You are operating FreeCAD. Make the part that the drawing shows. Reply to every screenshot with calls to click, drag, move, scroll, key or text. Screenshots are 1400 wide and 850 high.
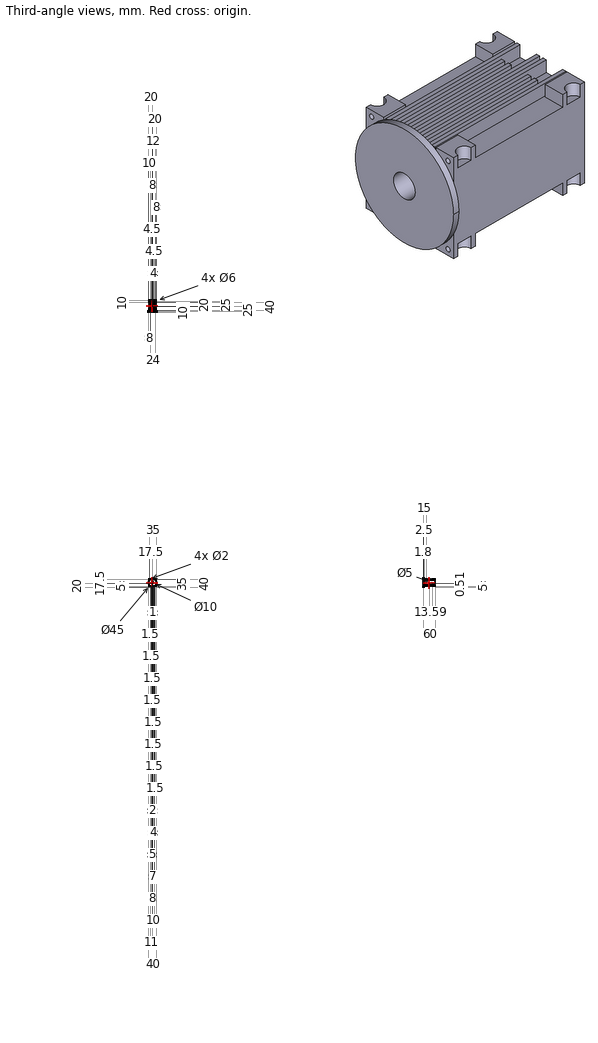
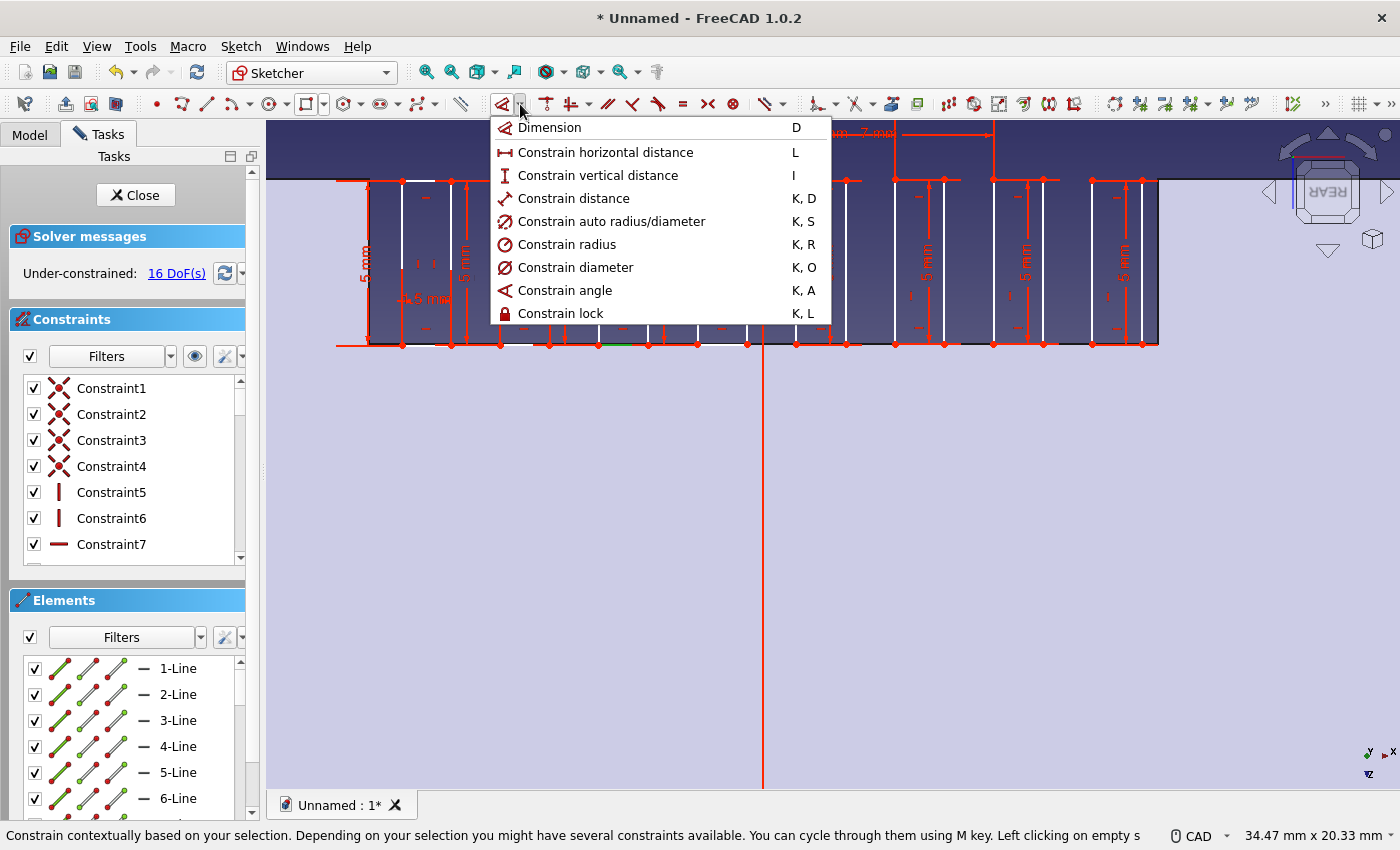
click(661, 152)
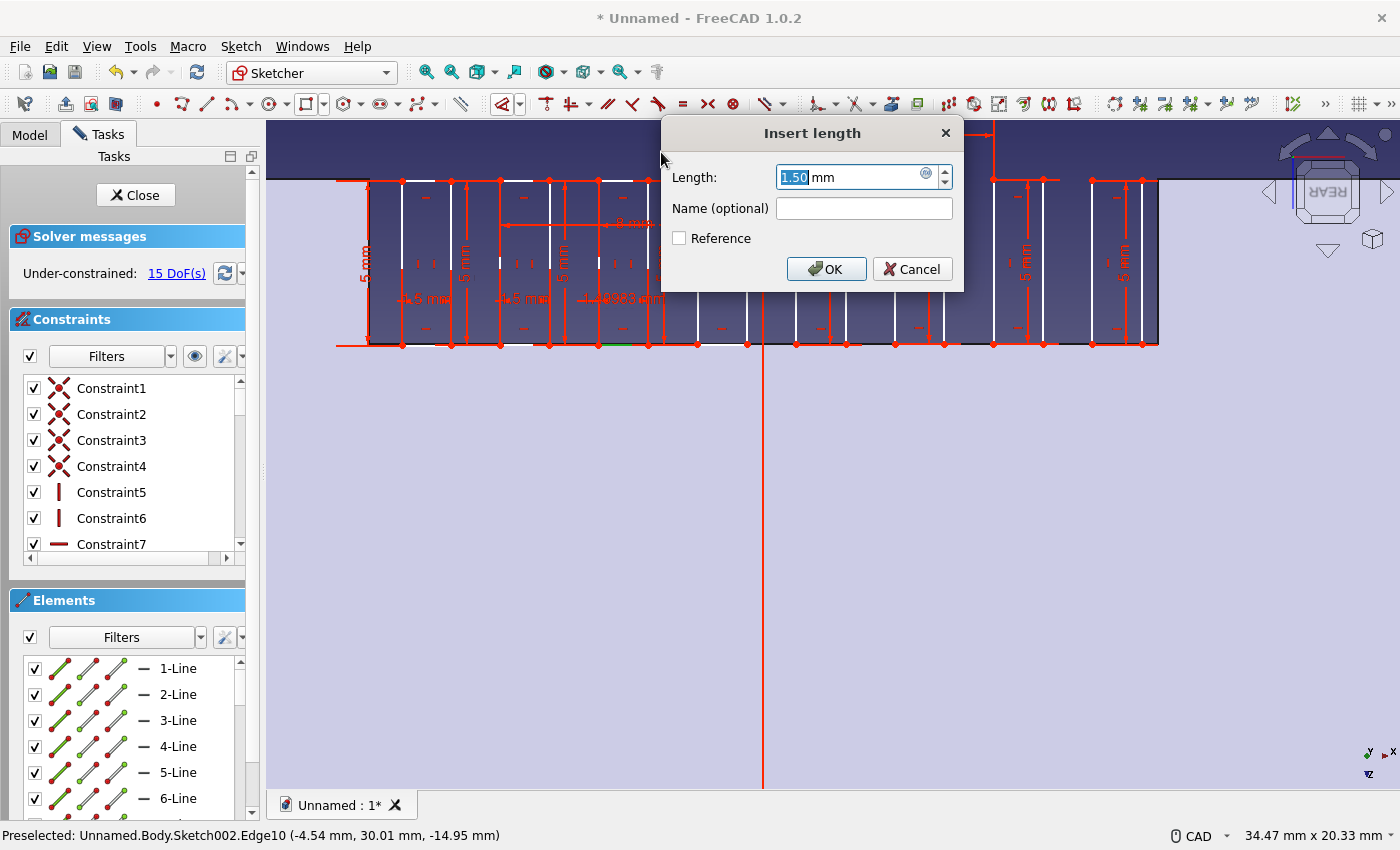
text(1.5)
key(Return)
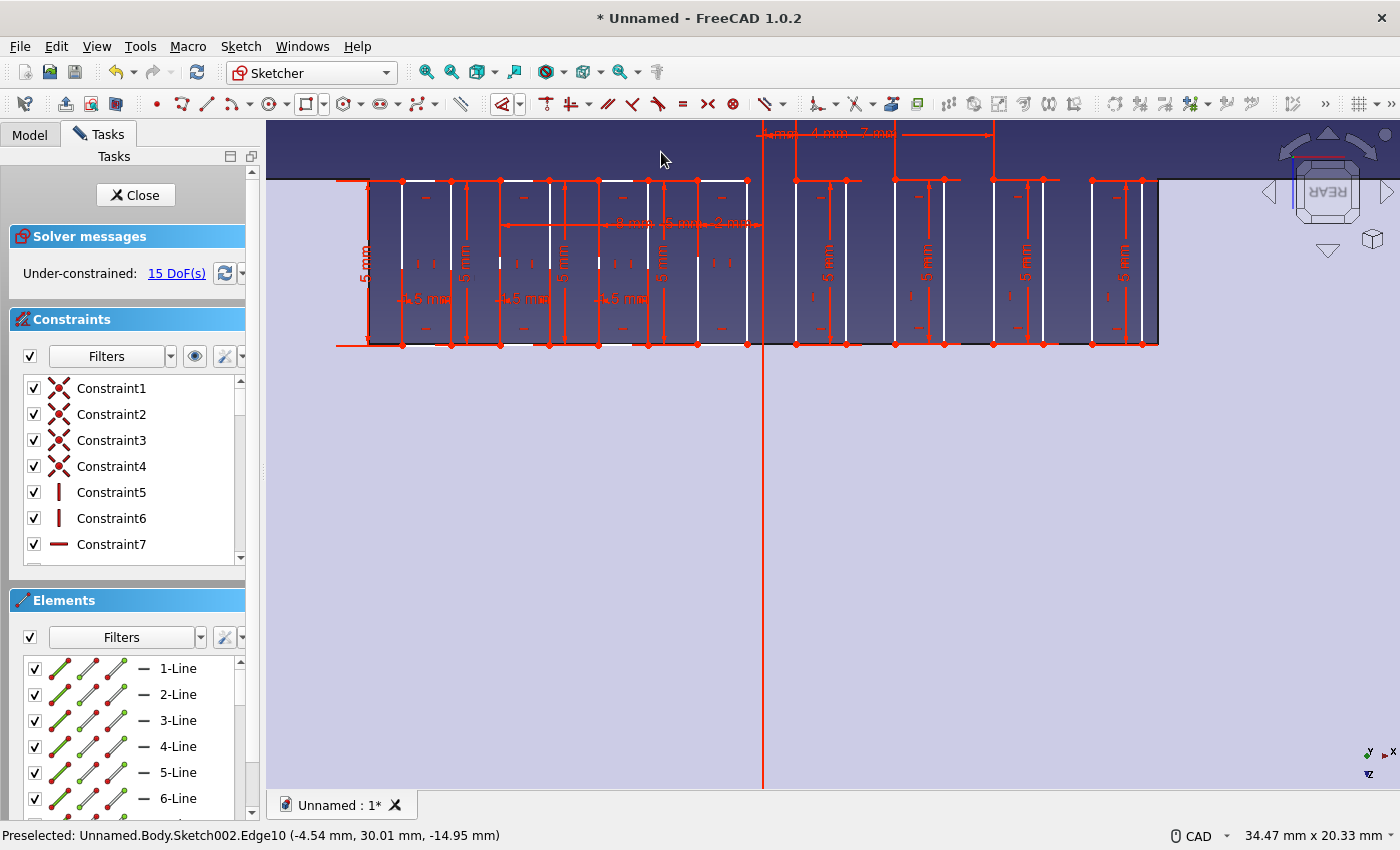
click(712, 345)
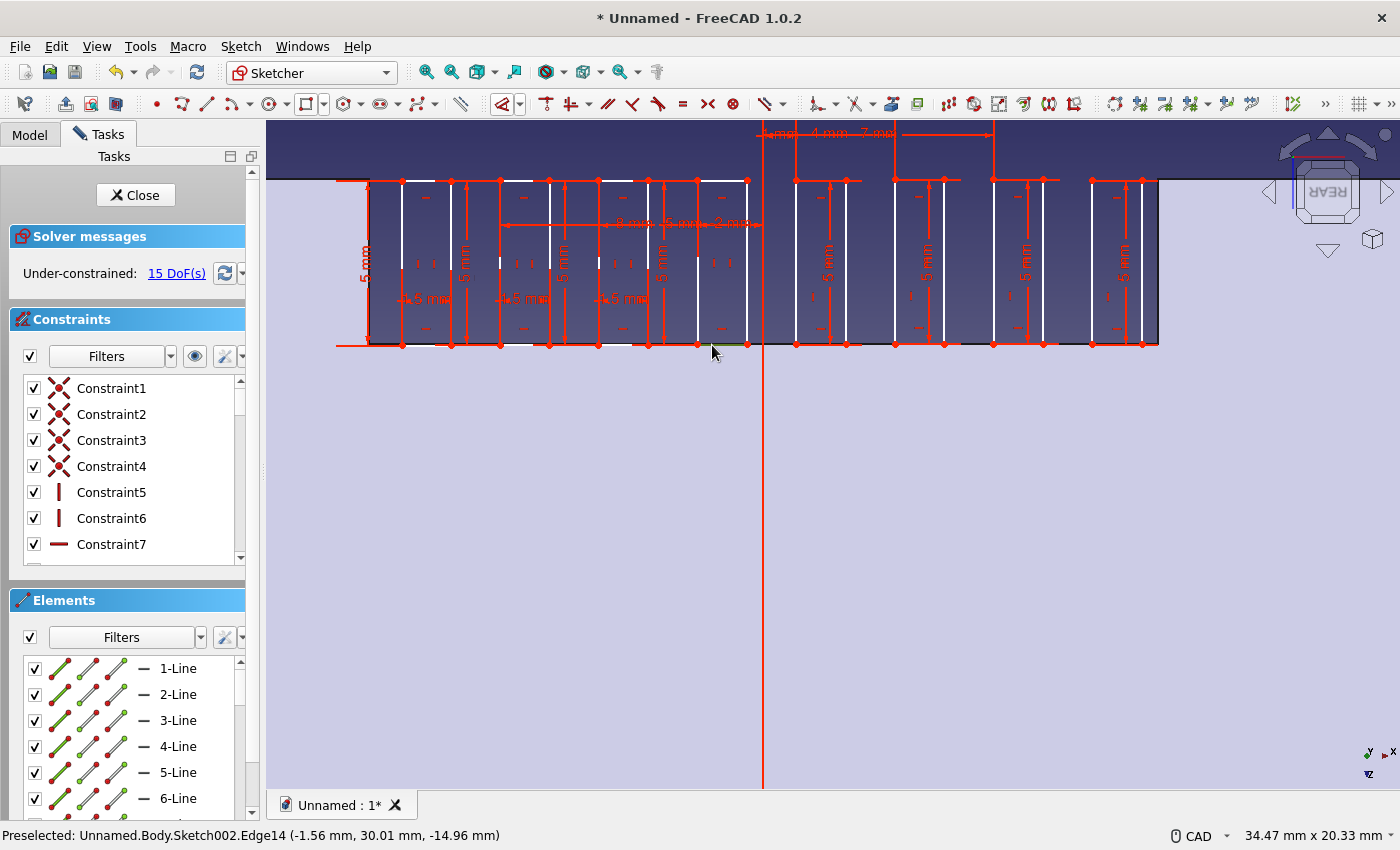
click(520, 104)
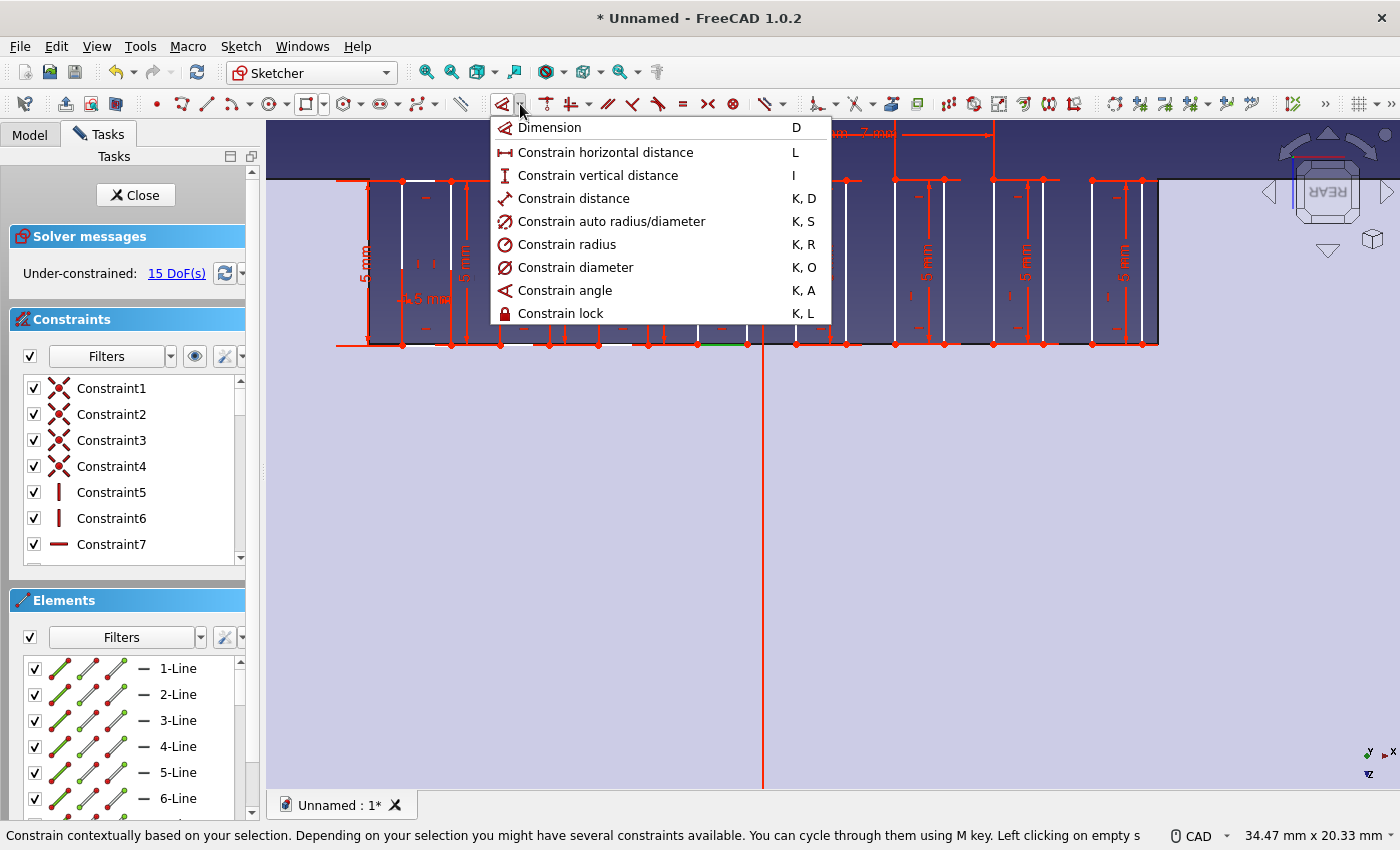
click(661, 152)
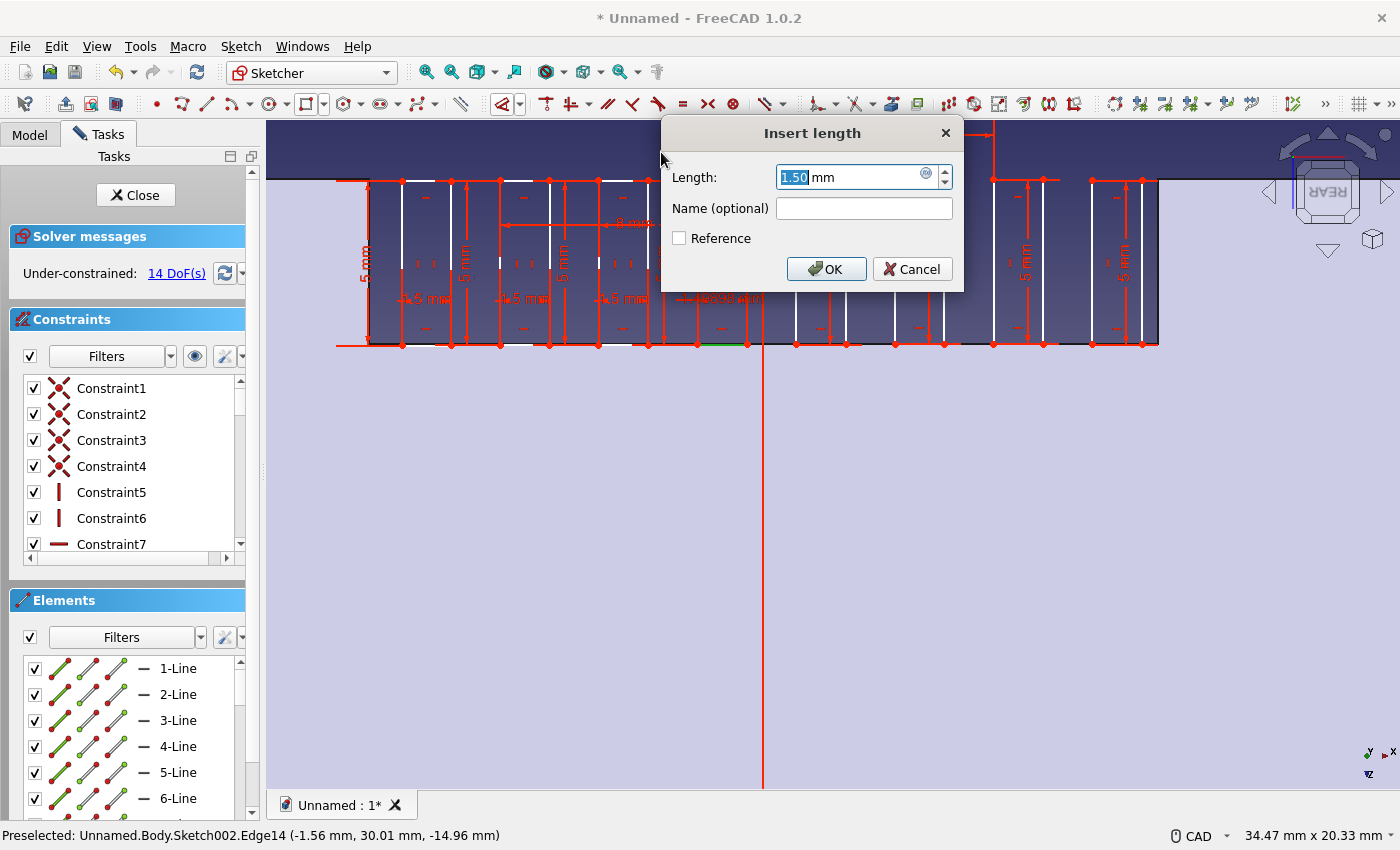
text(1.5)
key(Return)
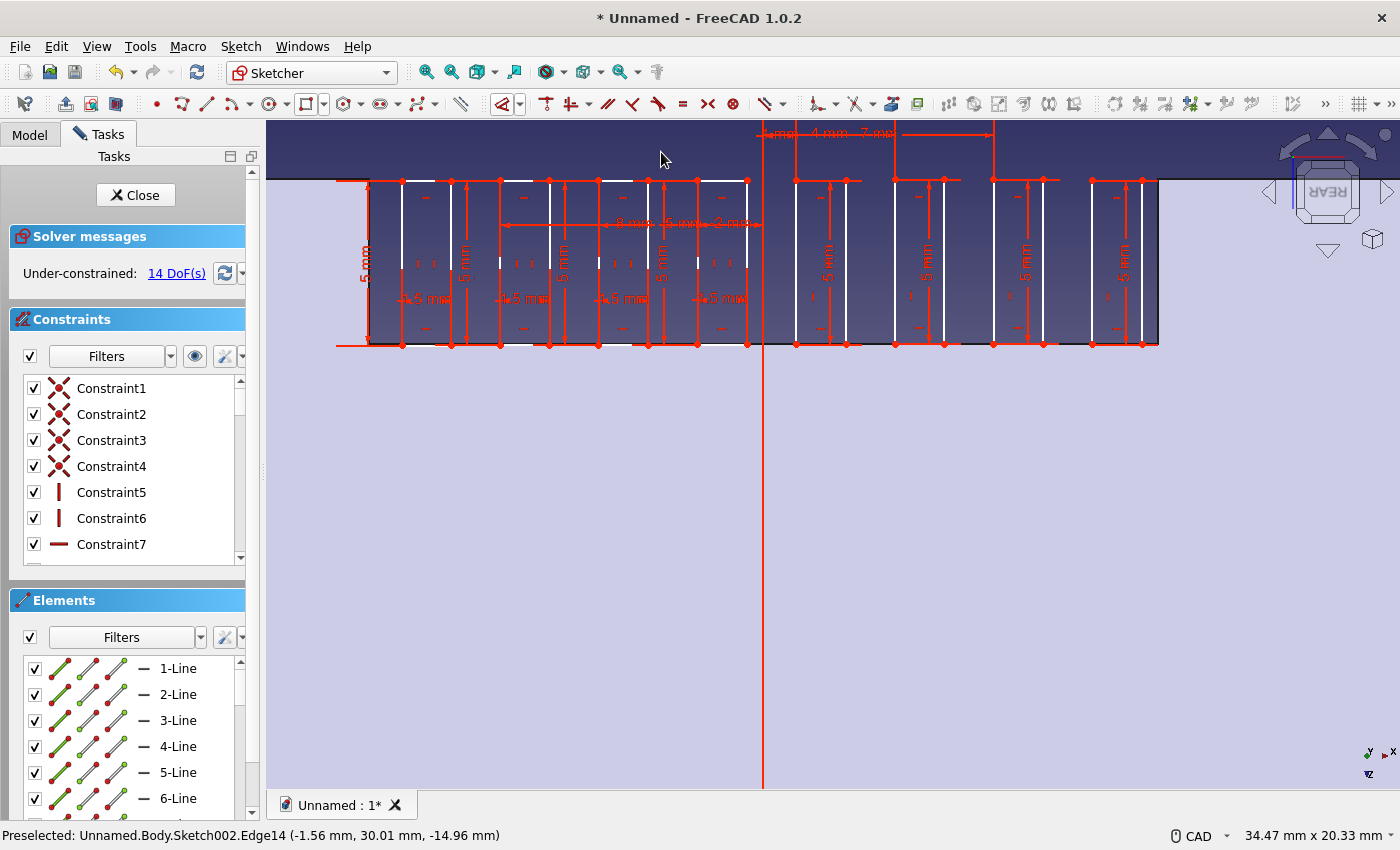
click(811, 345)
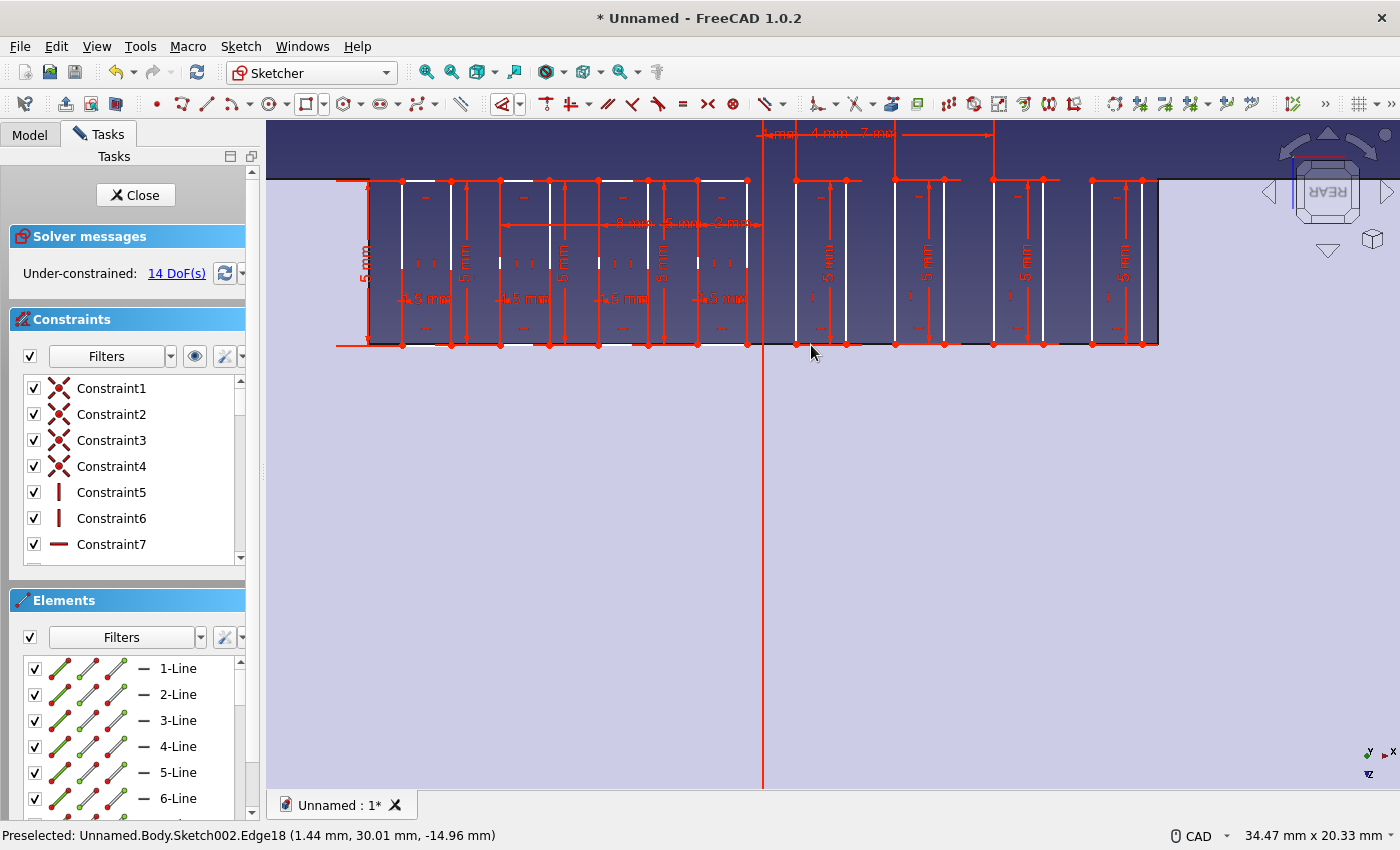
key(l)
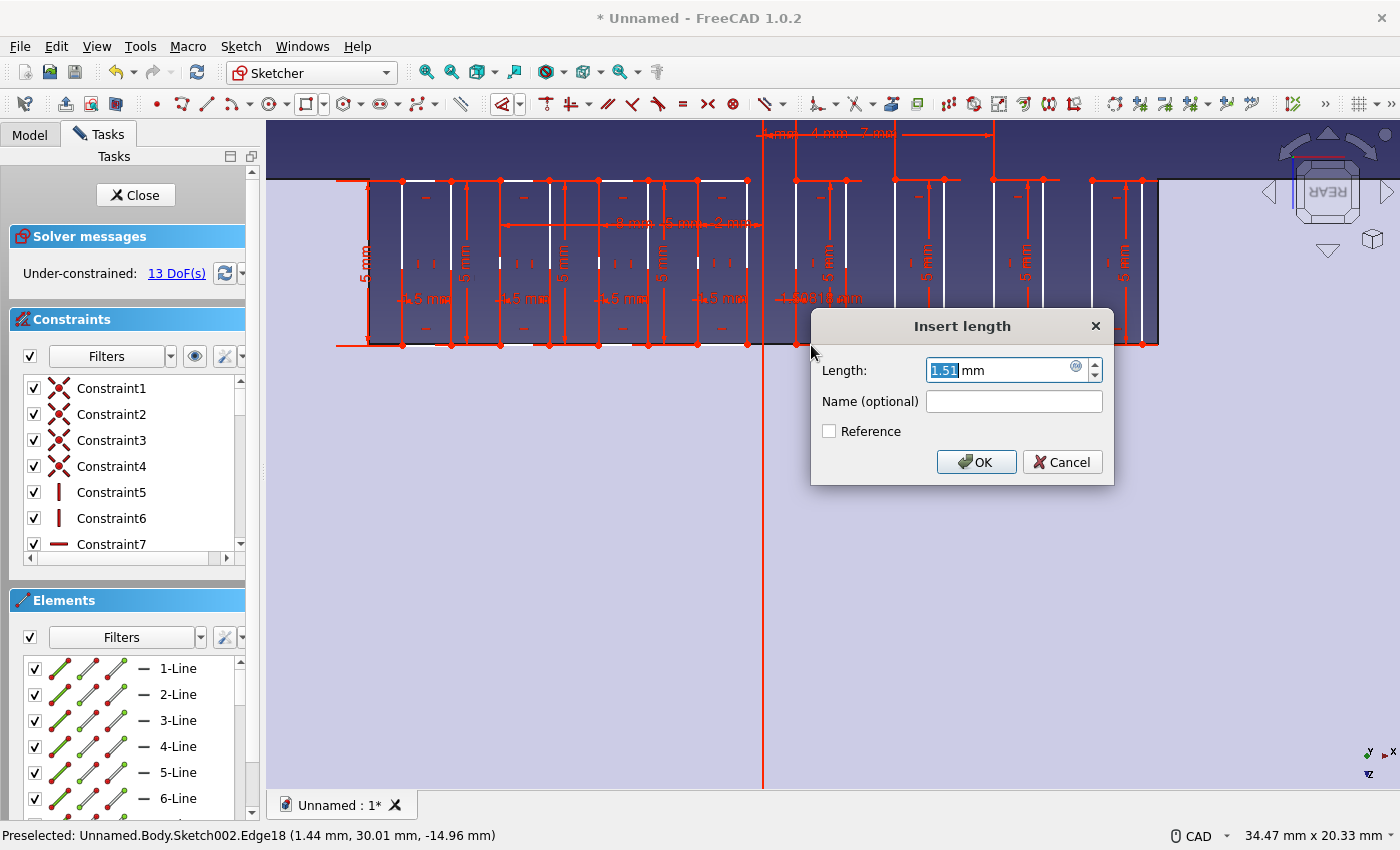
text(1.5)
key(Return)